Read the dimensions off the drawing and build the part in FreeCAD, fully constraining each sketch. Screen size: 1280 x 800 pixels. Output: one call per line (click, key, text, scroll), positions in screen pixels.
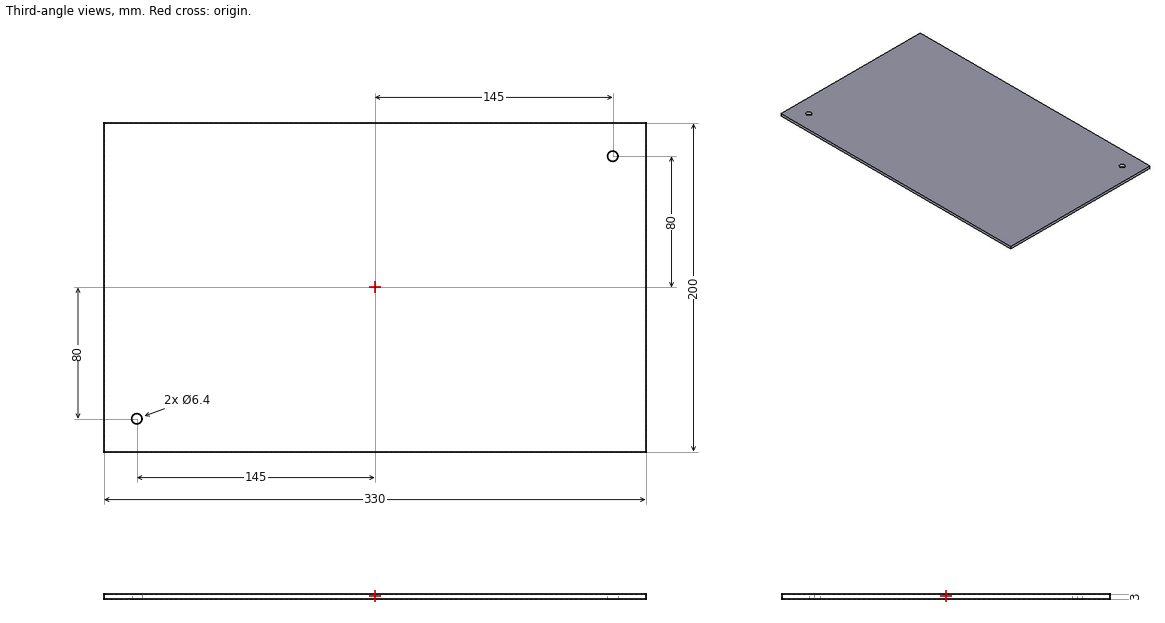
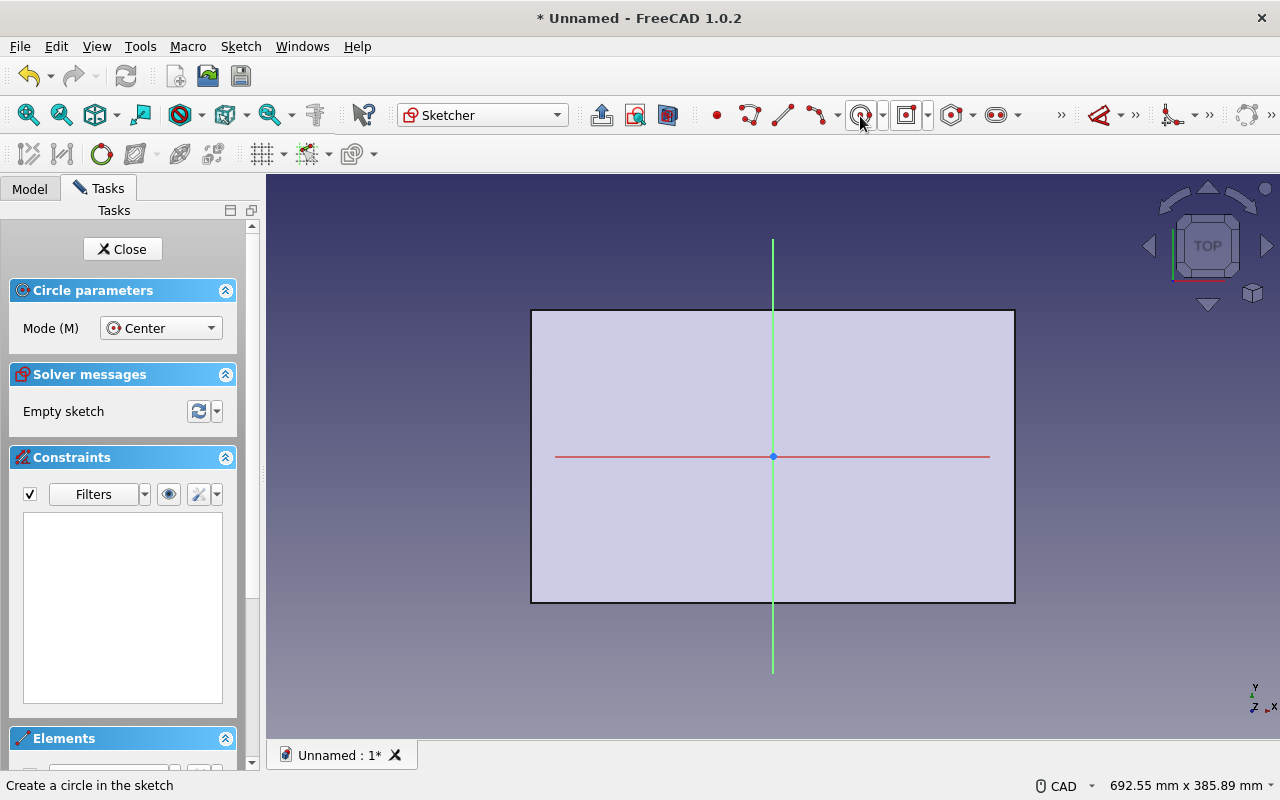
scroll(561, 574, up, 8)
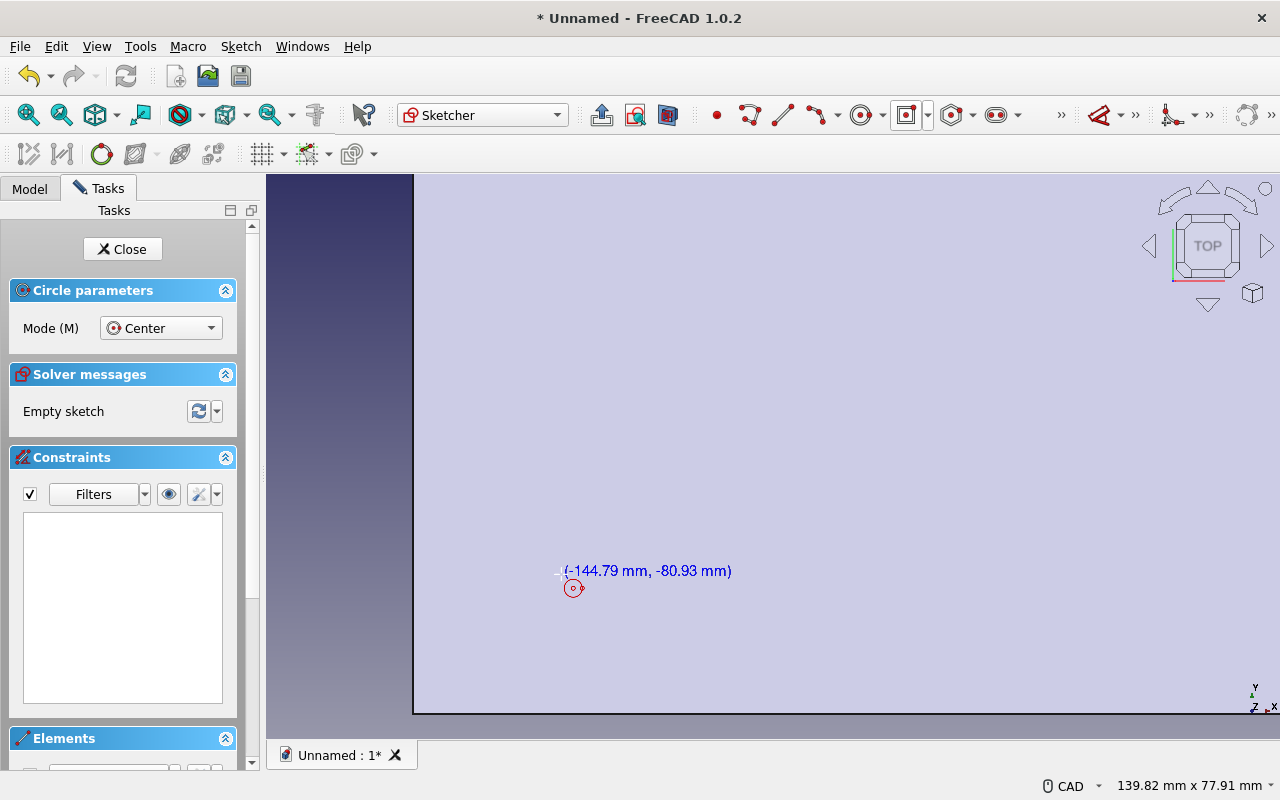
scroll(408, 609, down, 7)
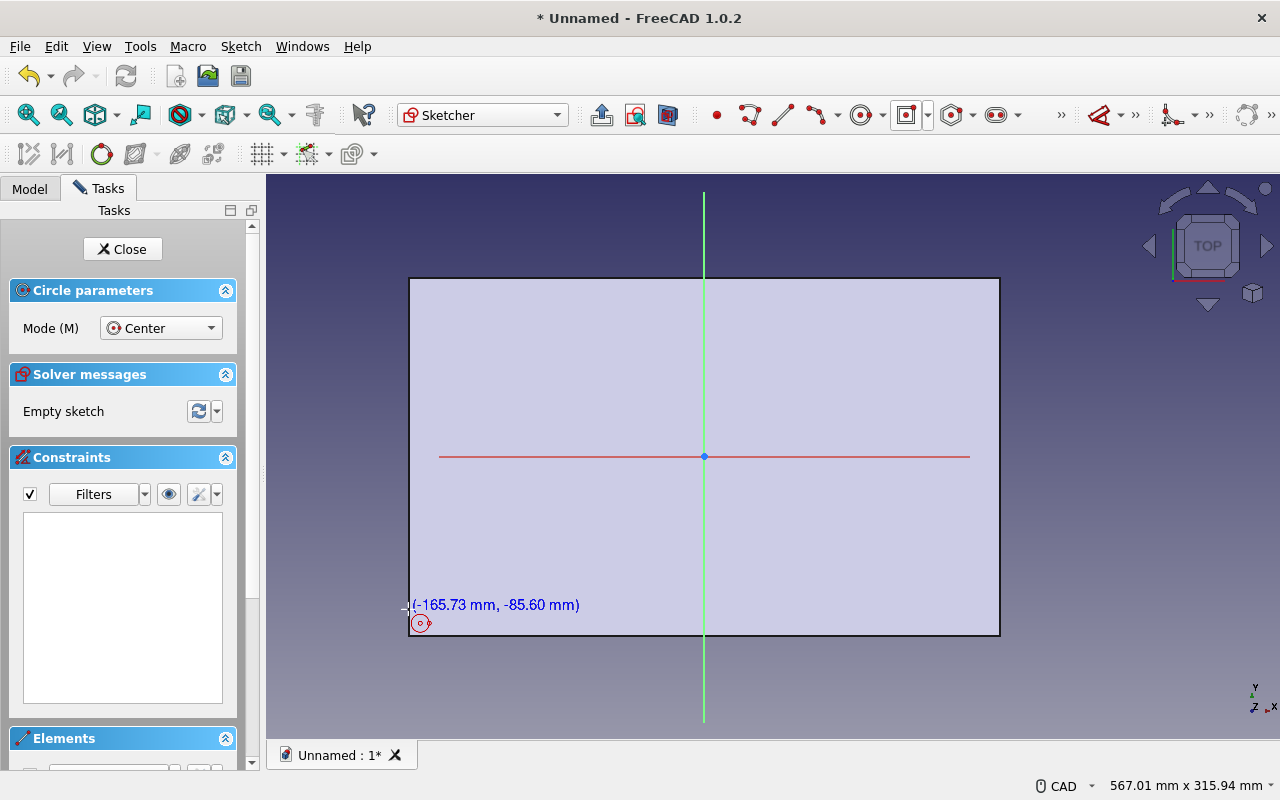
click(445, 600)
move(449, 596)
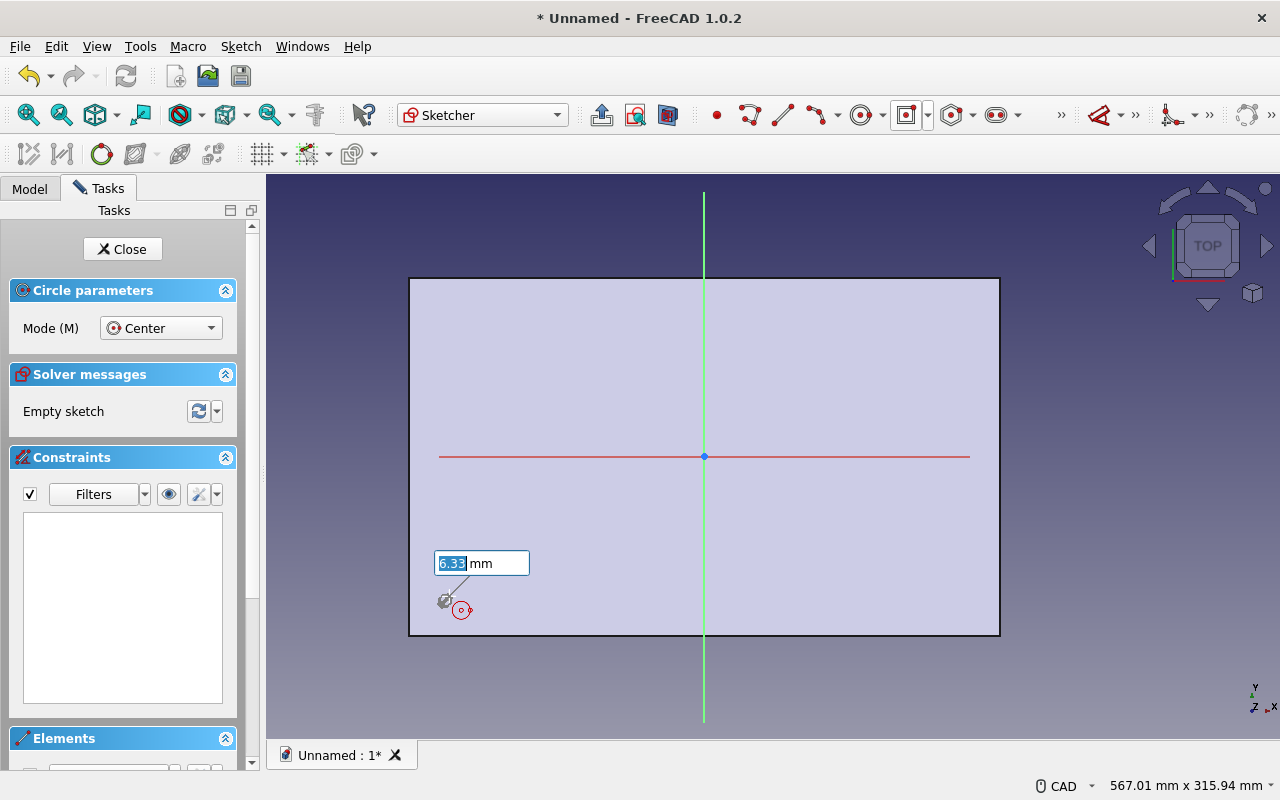
text(6.4)
key(Return)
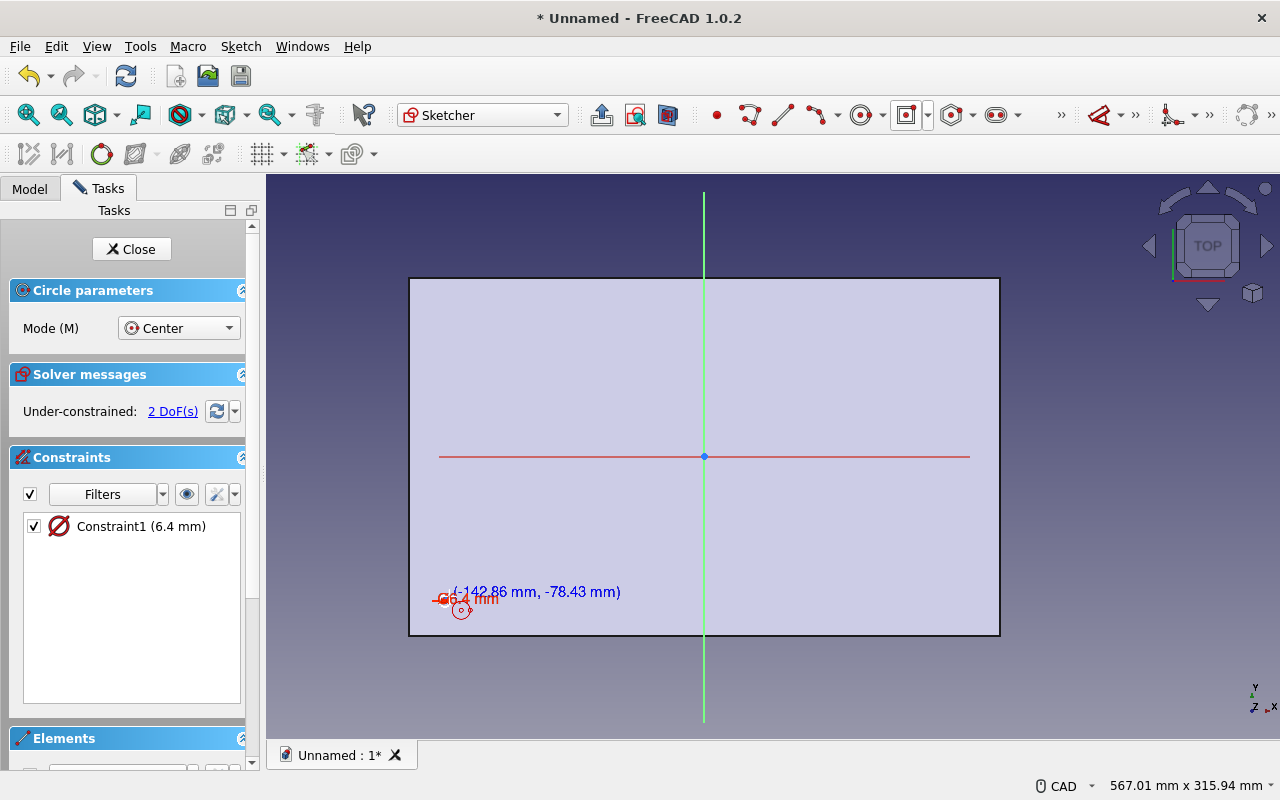
scroll(964, 314, up, 7)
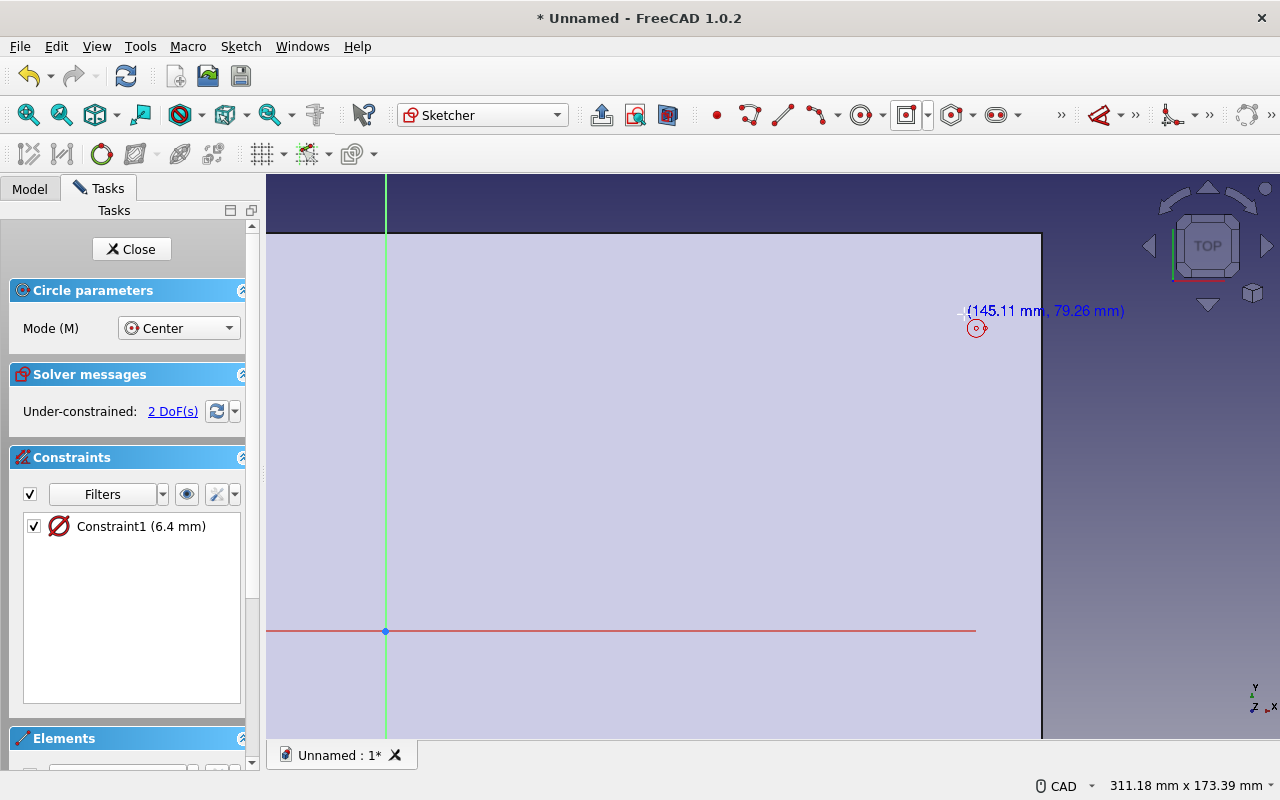
scroll(965, 314, down, 7)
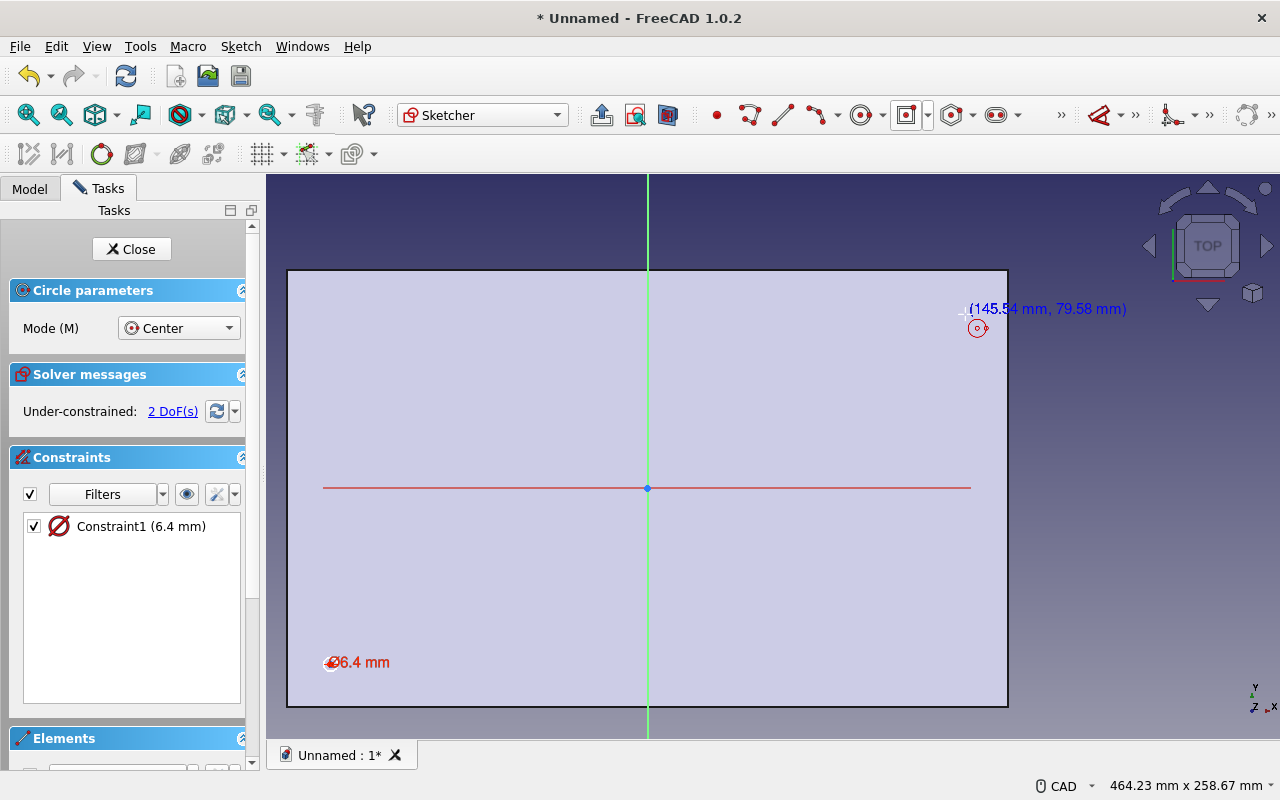
click(965, 314)
move(969, 310)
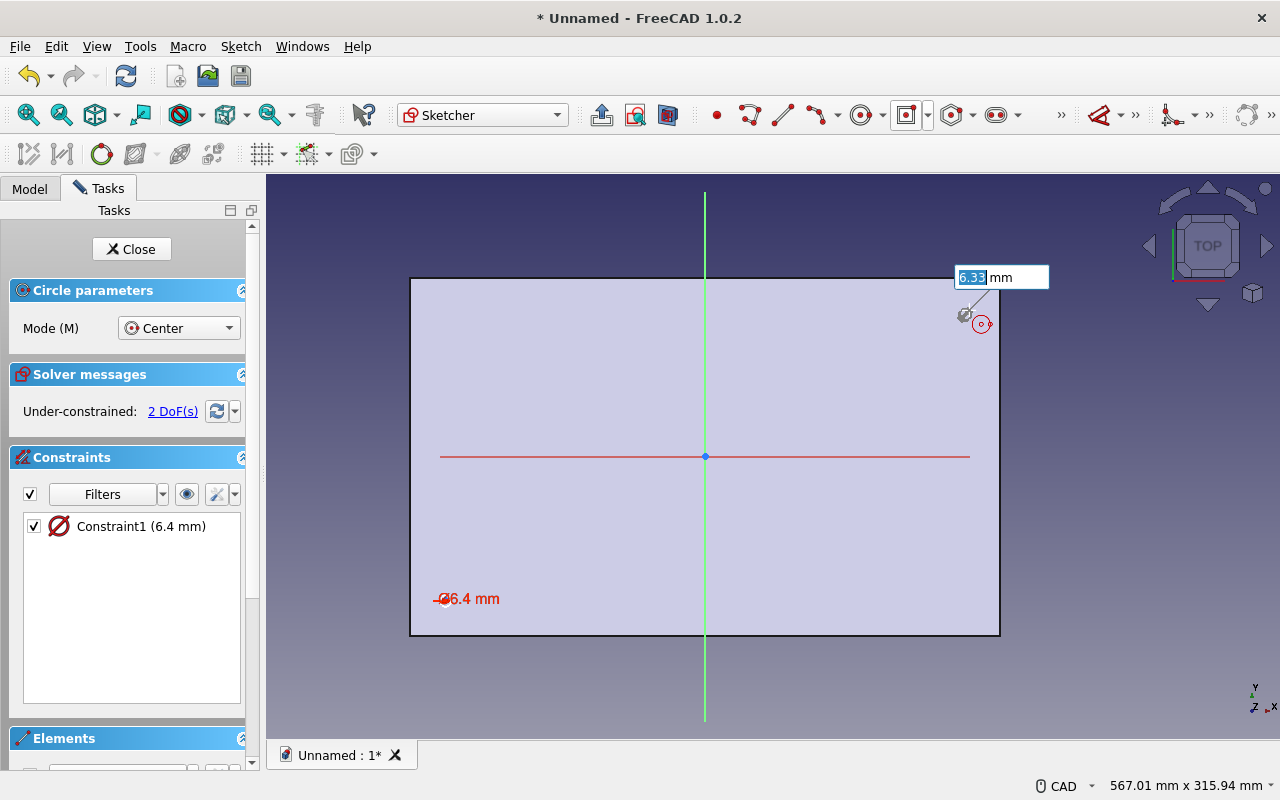
text(6.4)
key(Return)
key(Escape)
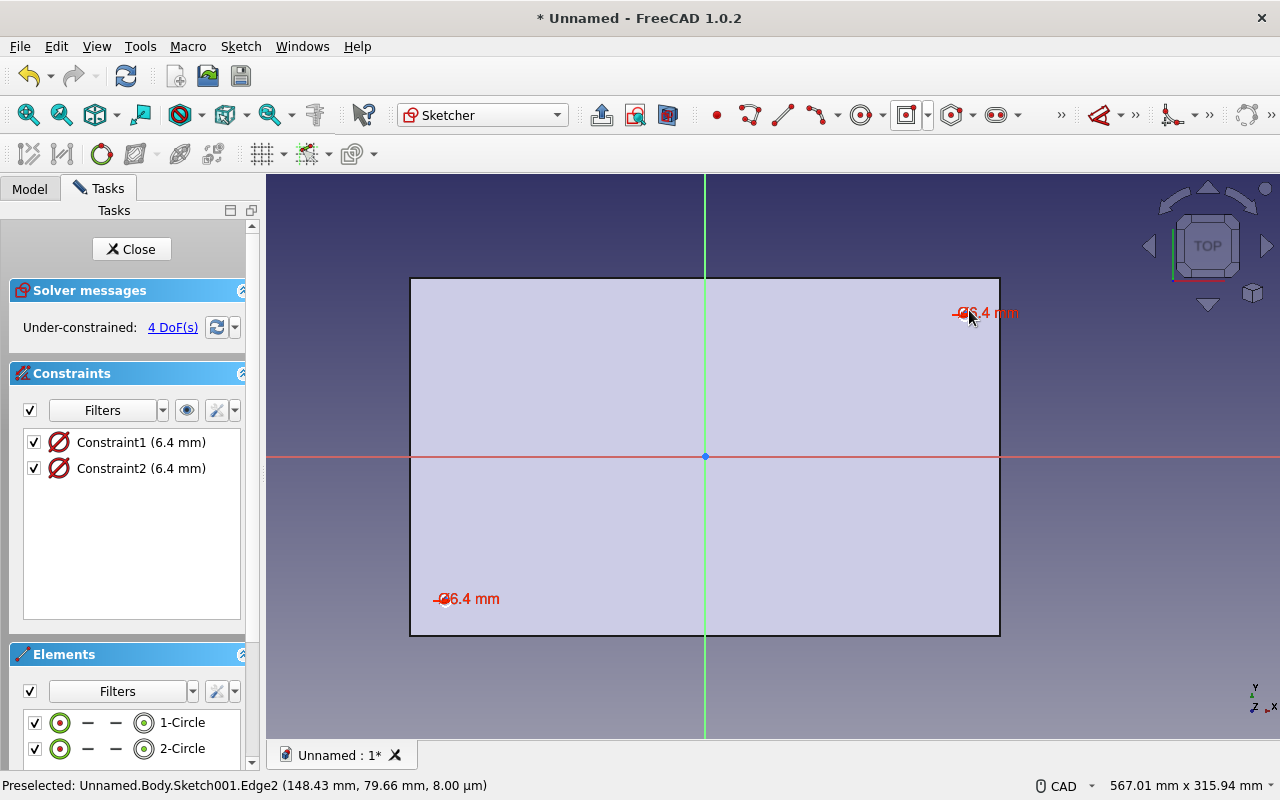
click(1098, 116)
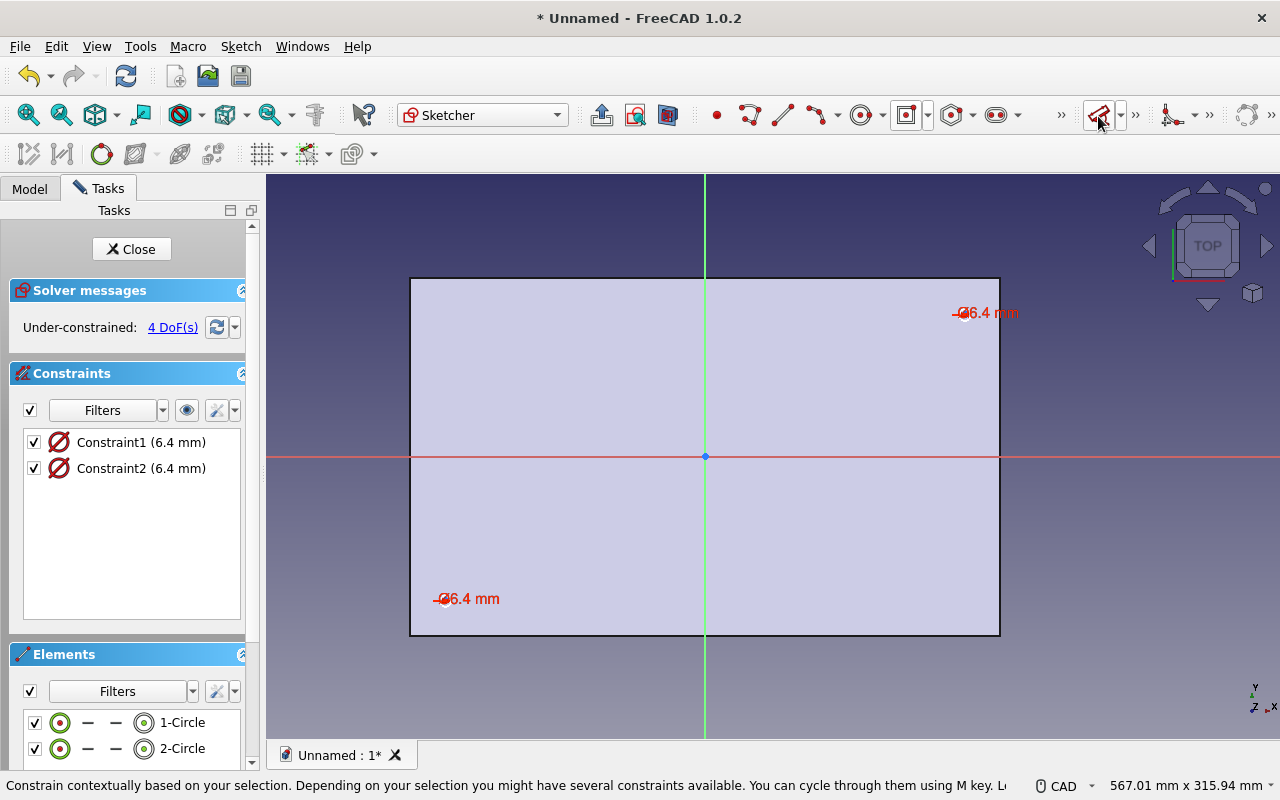
click(446, 601)
click(412, 529)